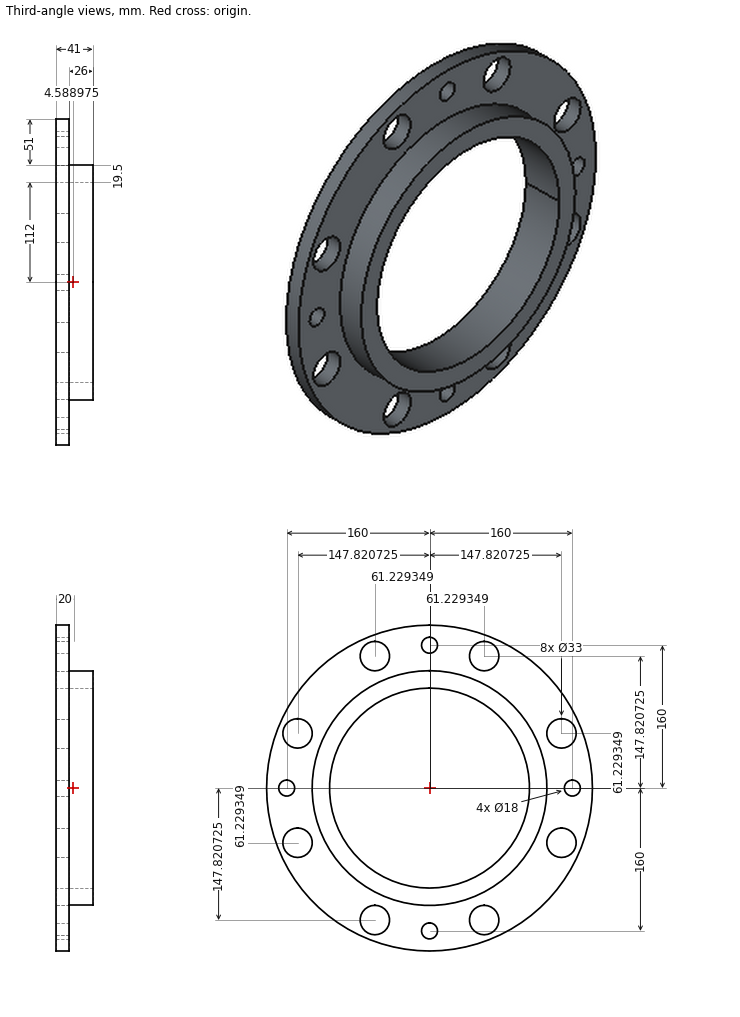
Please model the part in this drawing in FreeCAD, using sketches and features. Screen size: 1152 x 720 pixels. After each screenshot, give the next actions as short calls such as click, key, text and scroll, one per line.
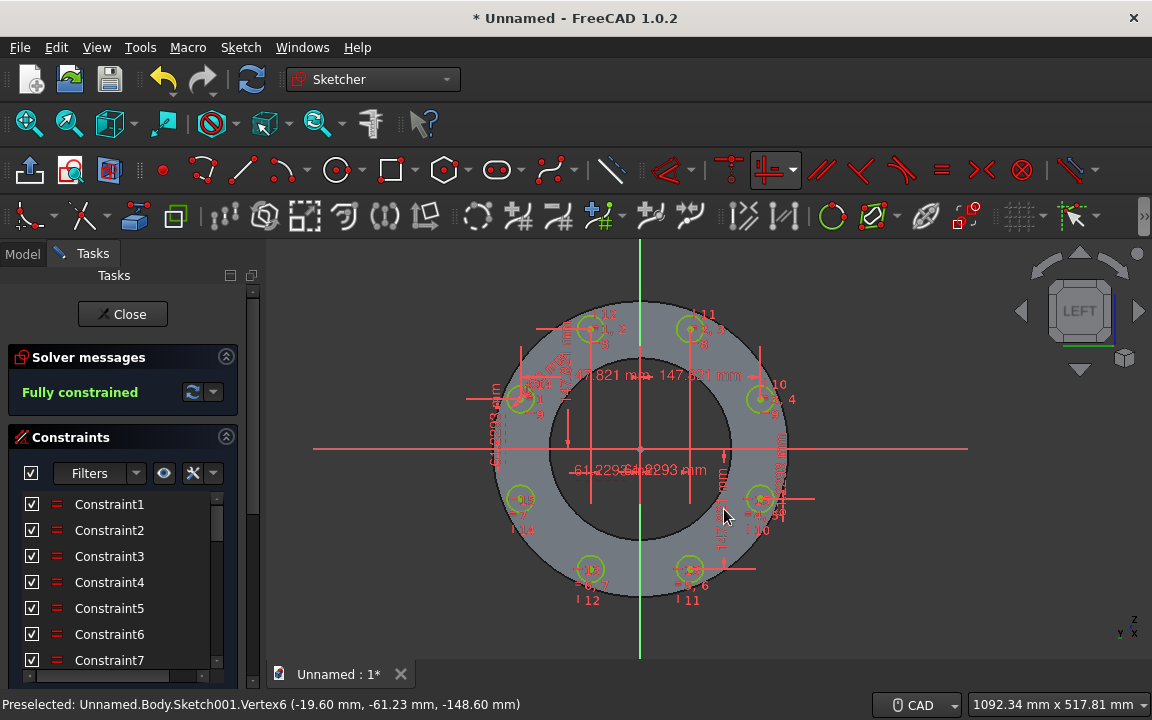
click(123, 314)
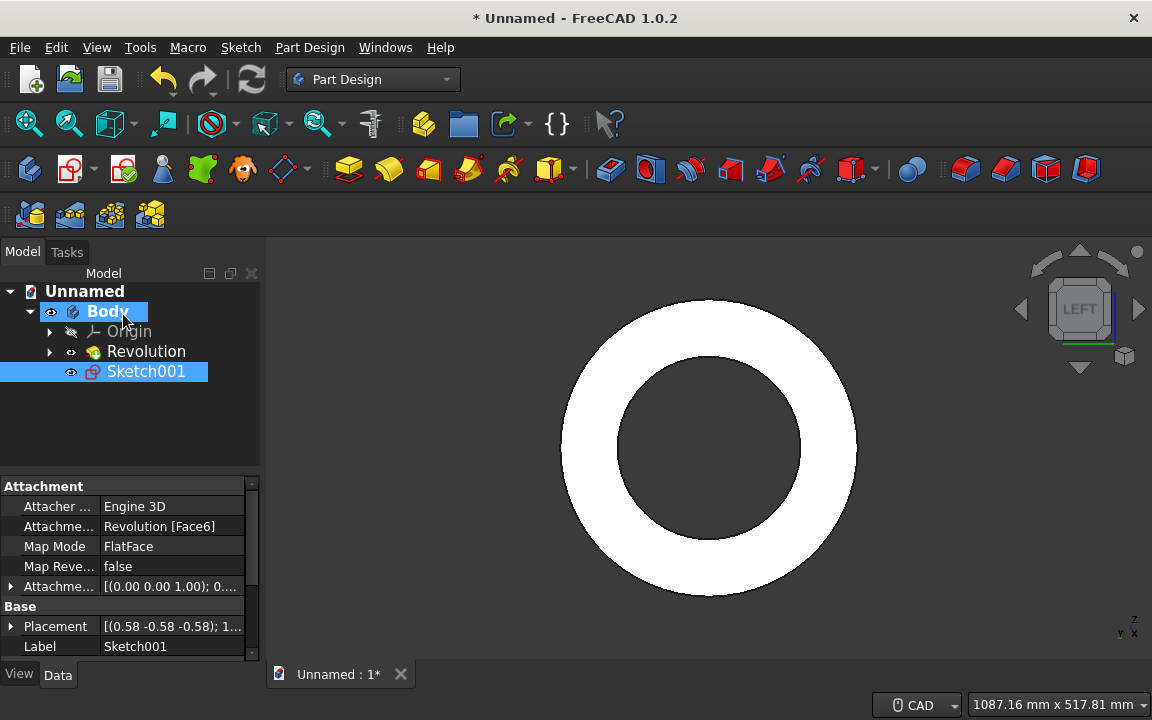
click(612, 170)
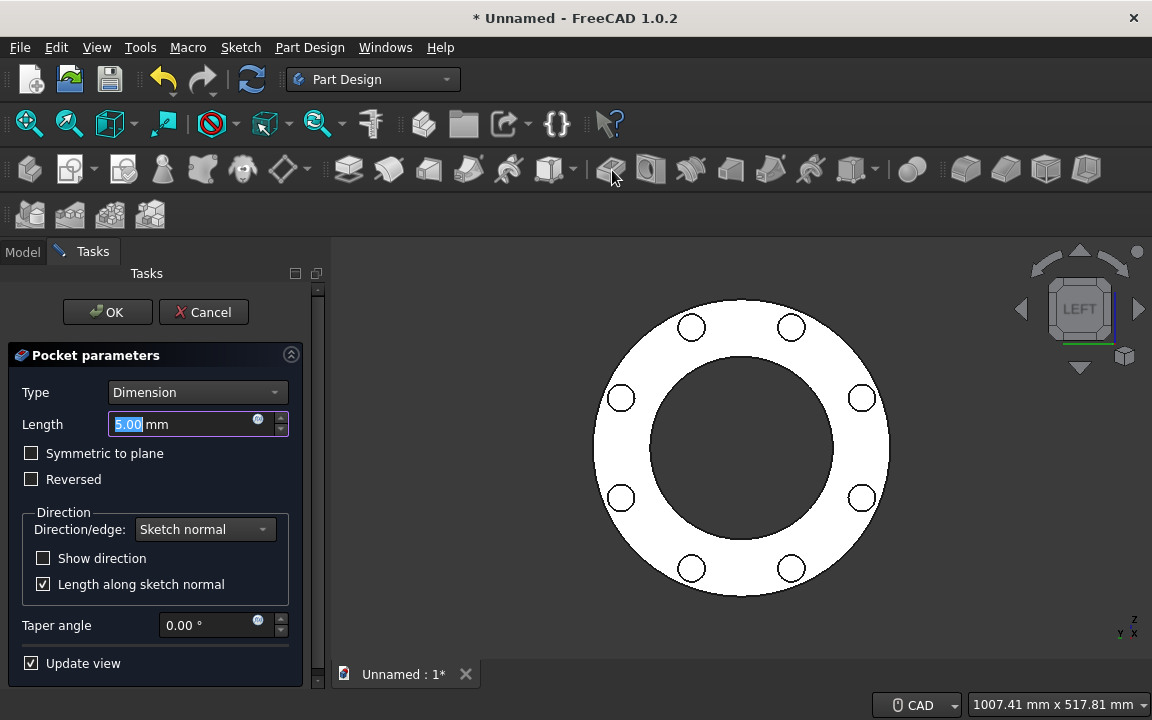
text(20)
key(Tab)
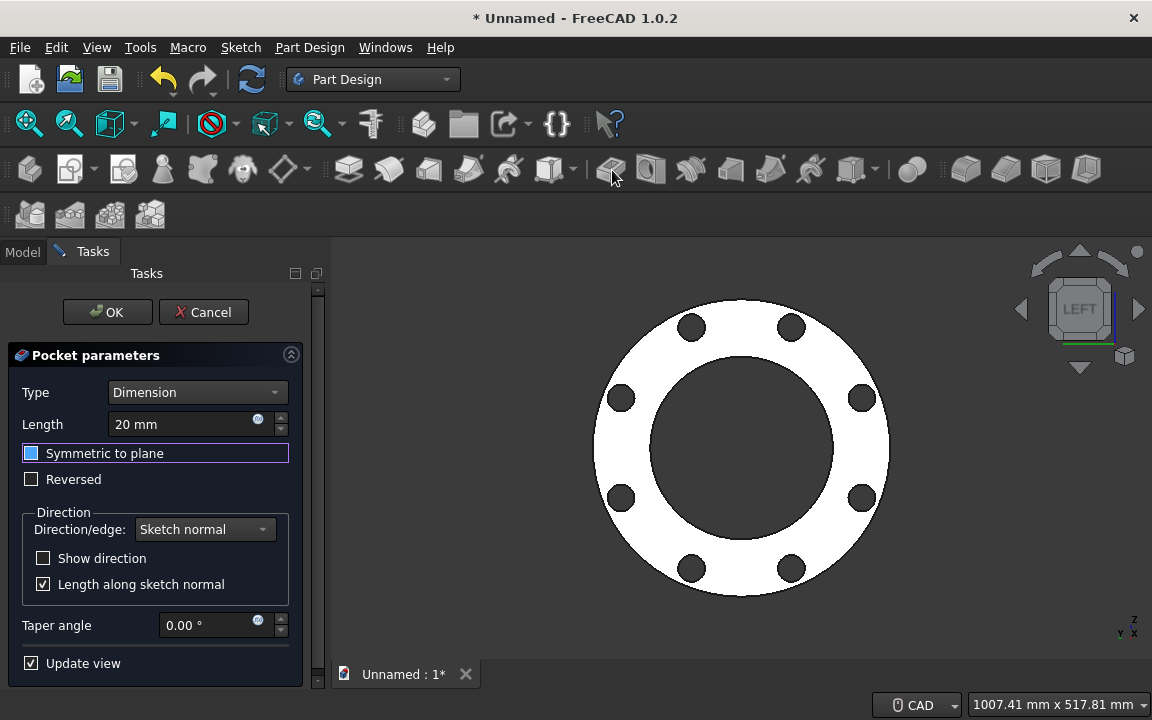
click(108, 312)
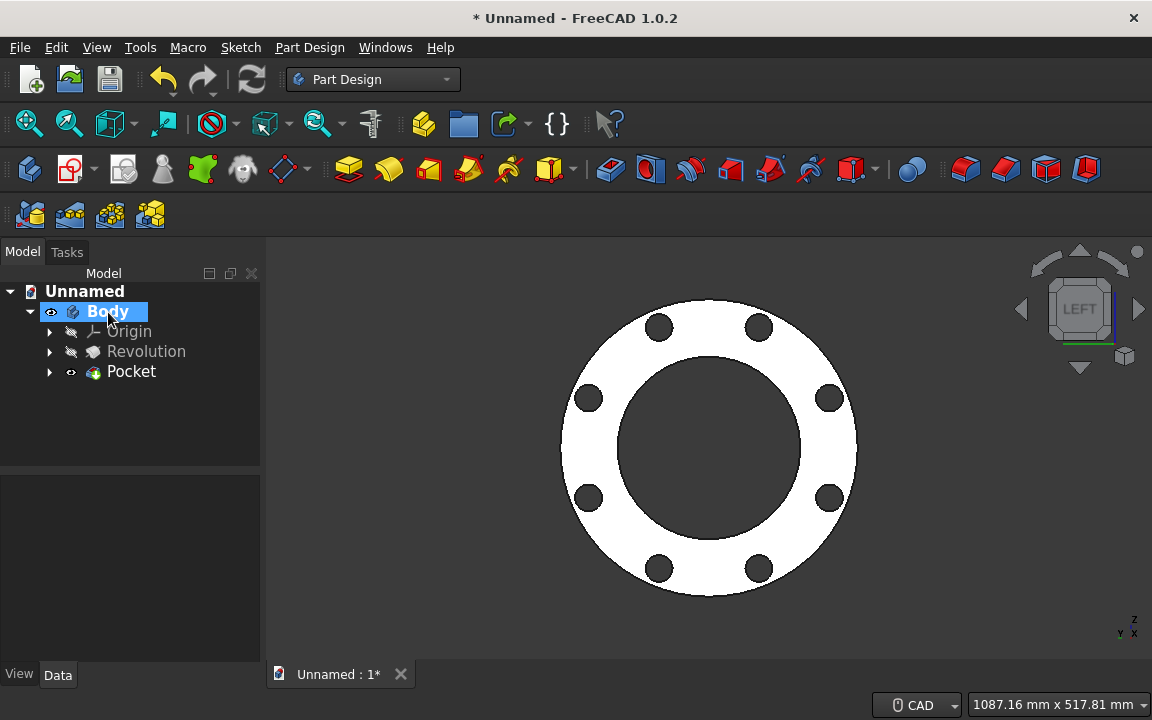
click(624, 362)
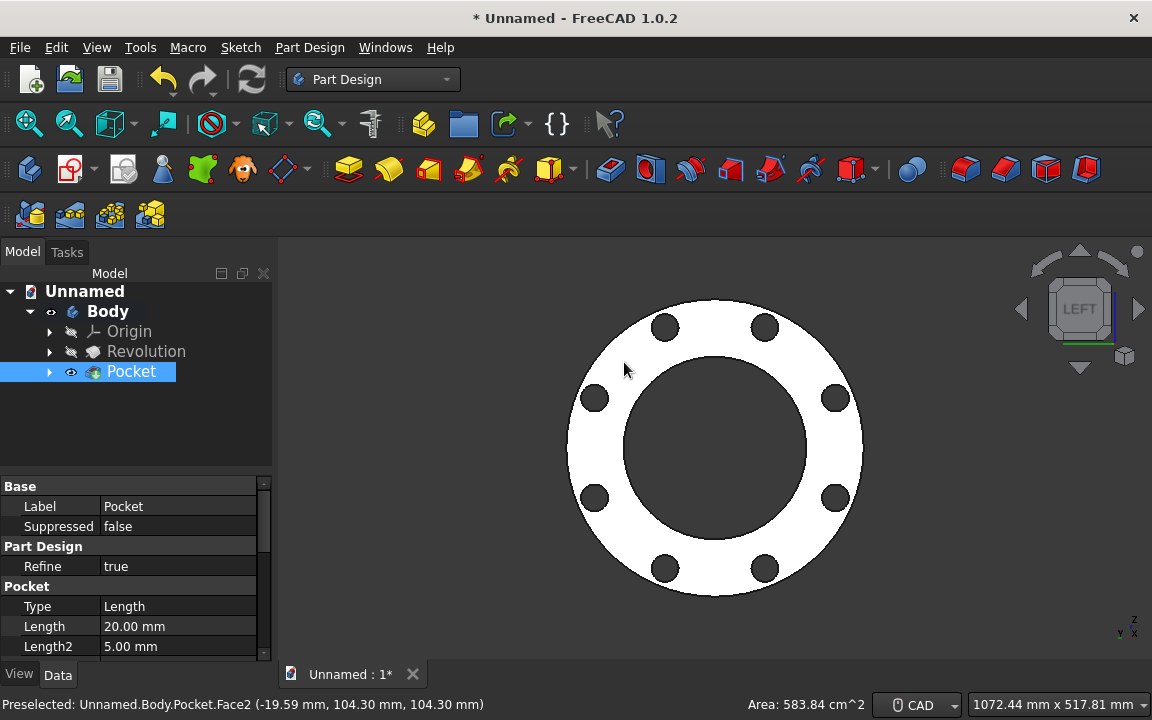
click(70, 170)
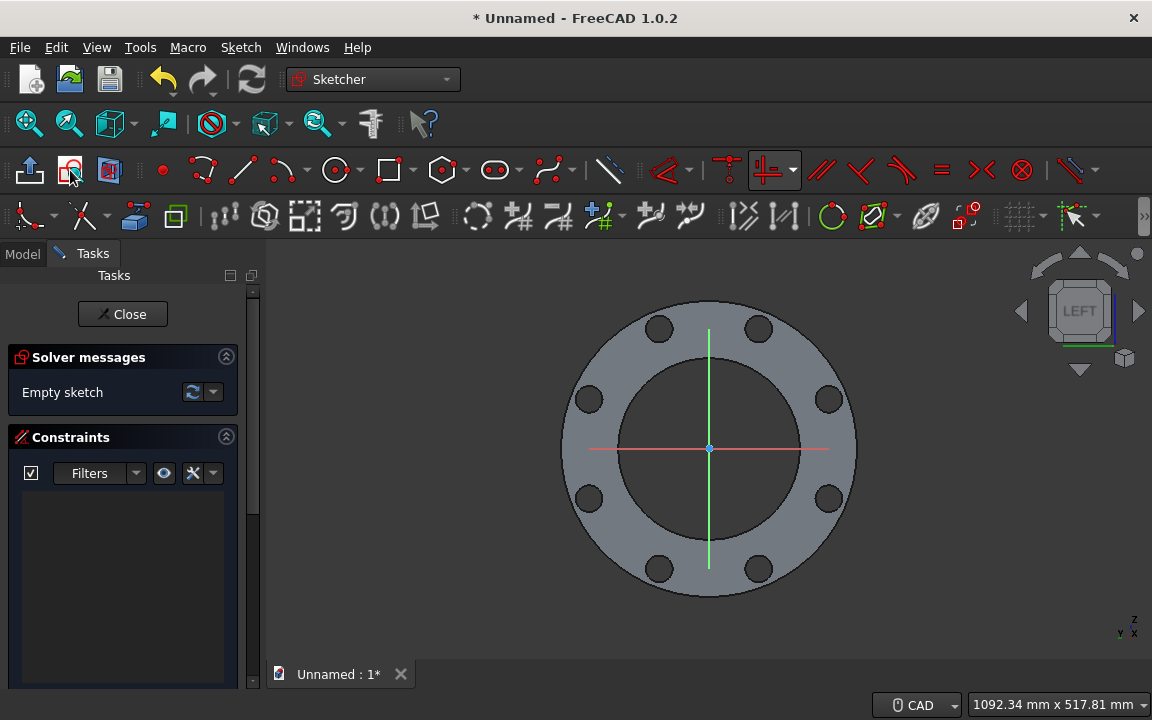
click(336, 170)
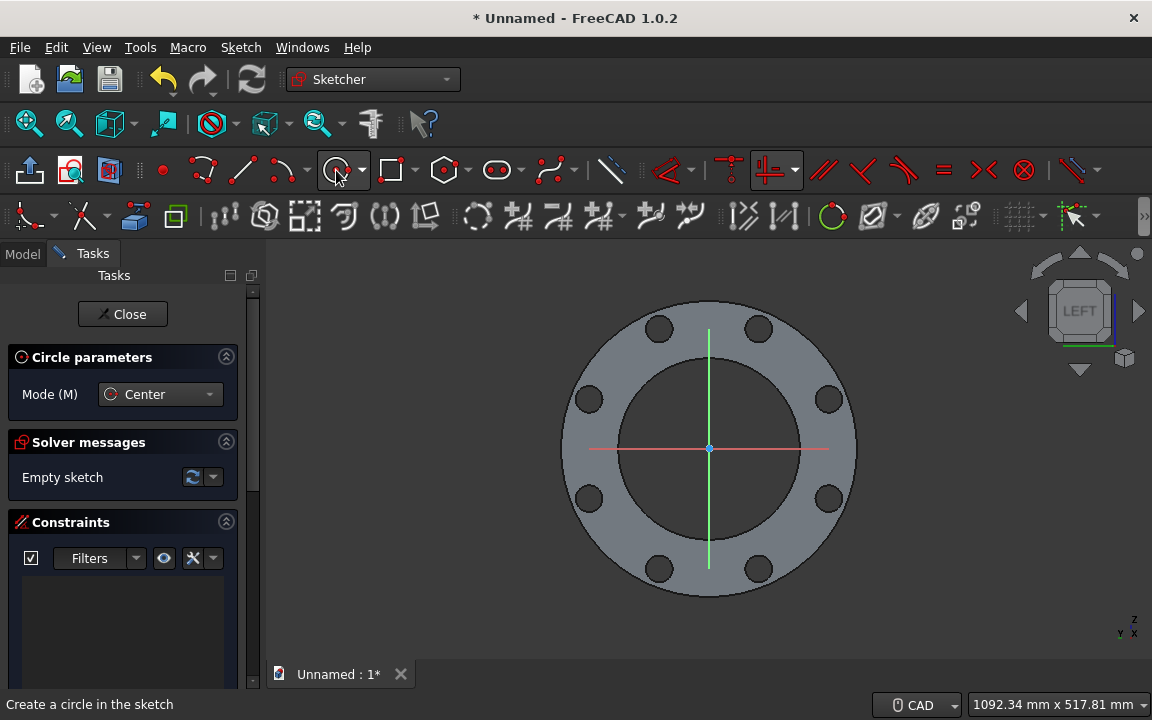
scroll(579, 449, up, 6)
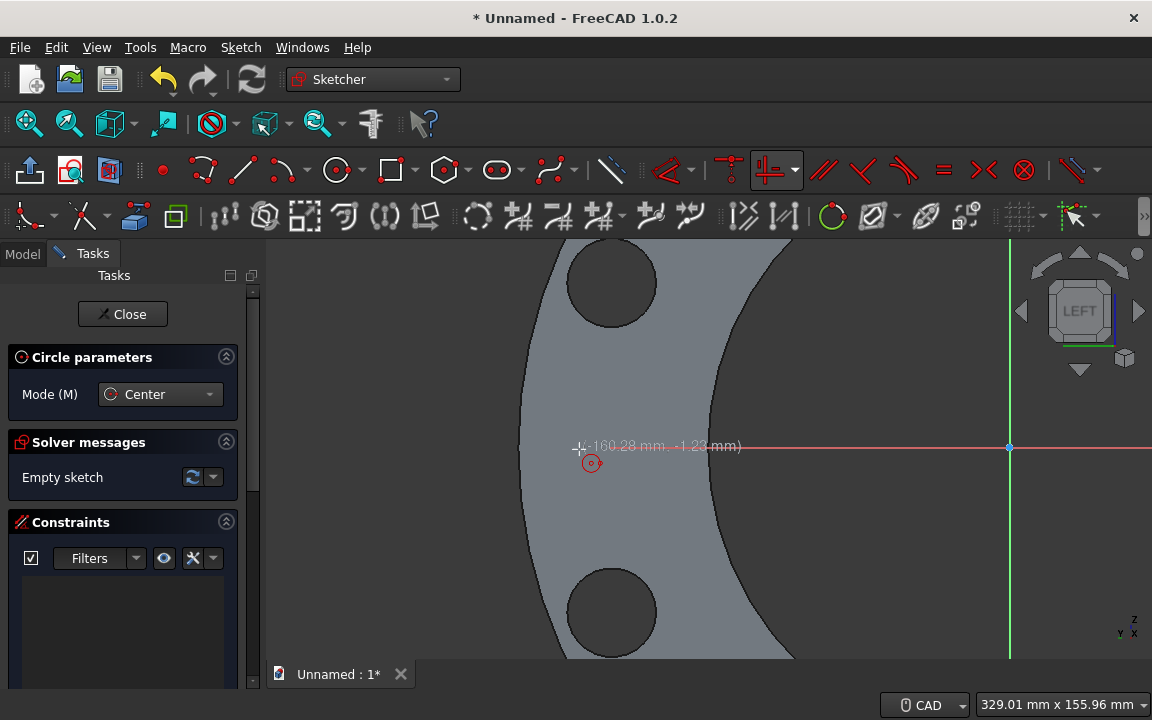
click(579, 448)
click(596, 431)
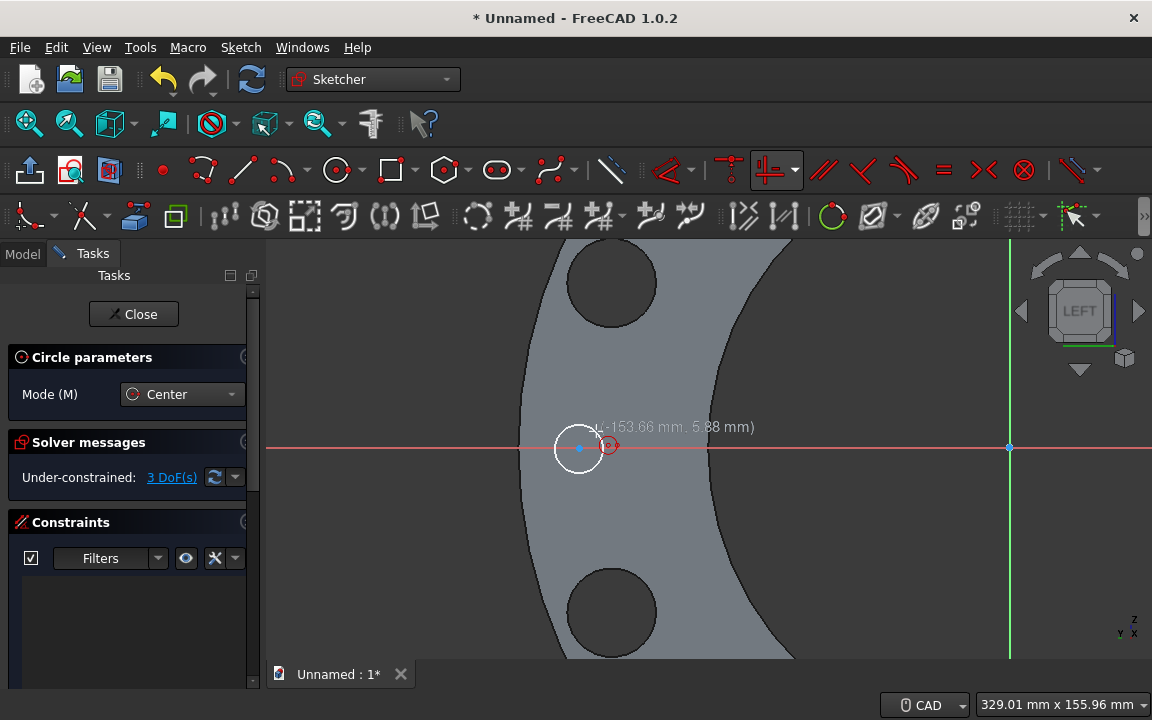
scroll(481, 450, down, 6)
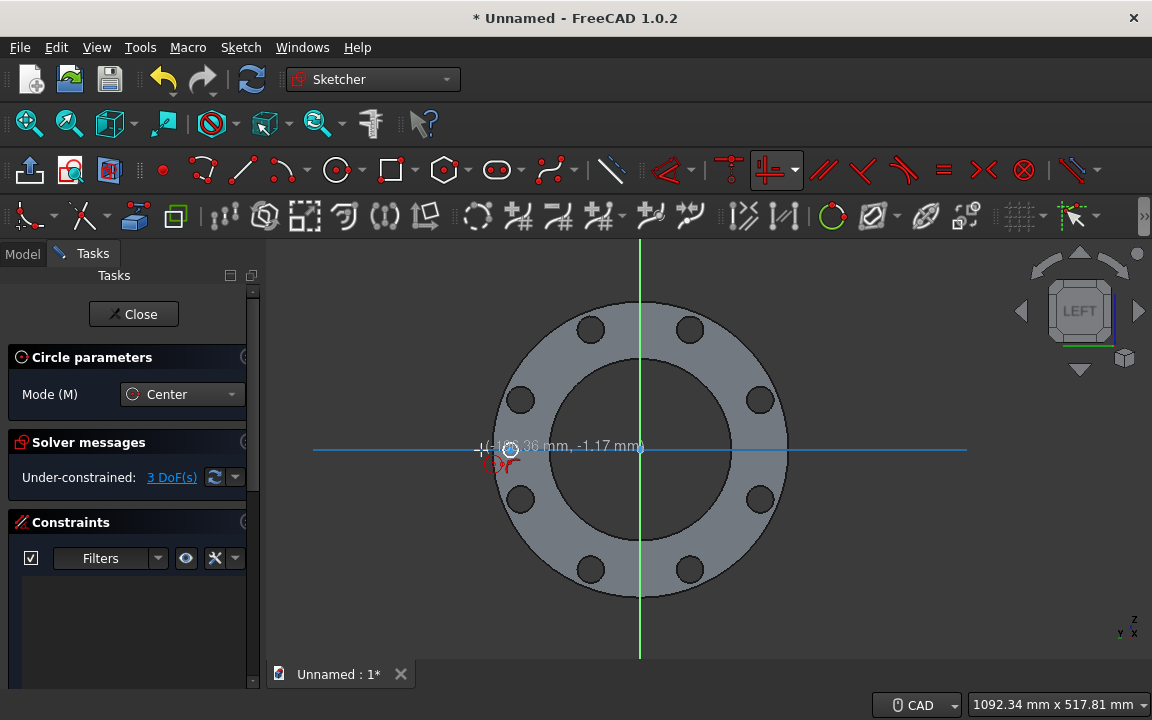
scroll(640, 320, up, 6)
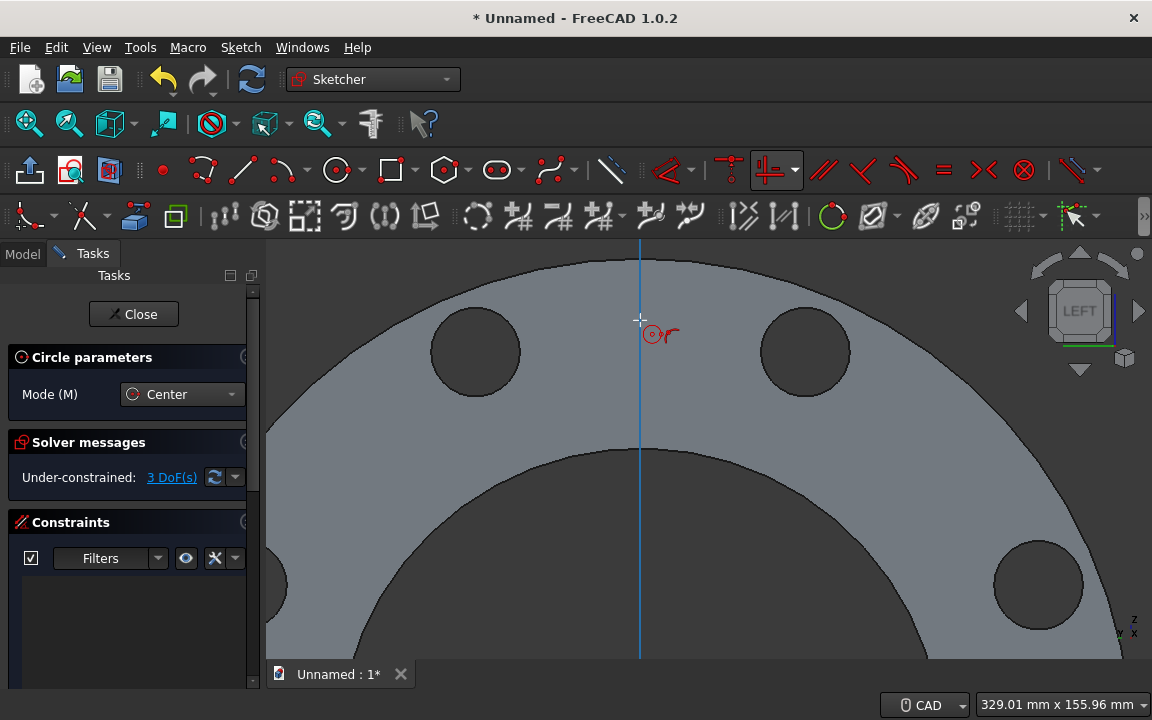
click(640, 319)
click(658, 302)